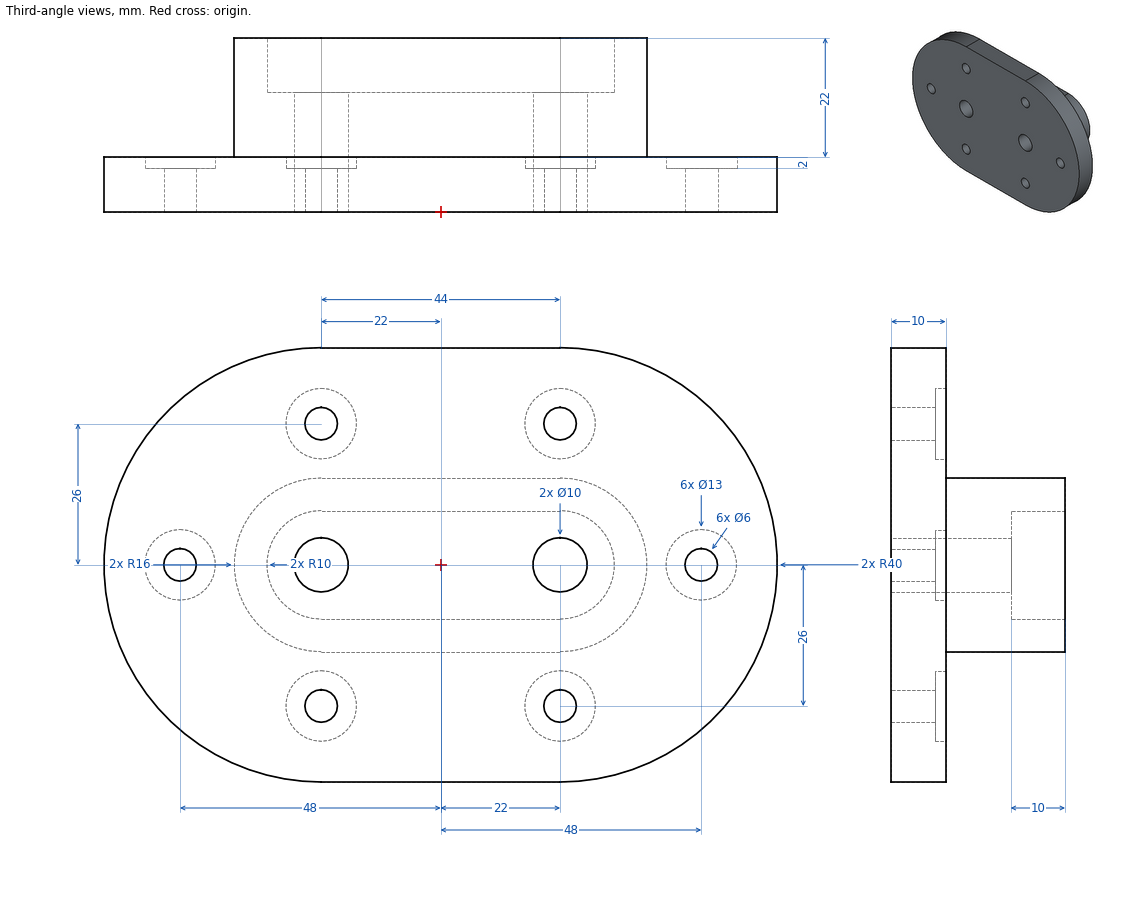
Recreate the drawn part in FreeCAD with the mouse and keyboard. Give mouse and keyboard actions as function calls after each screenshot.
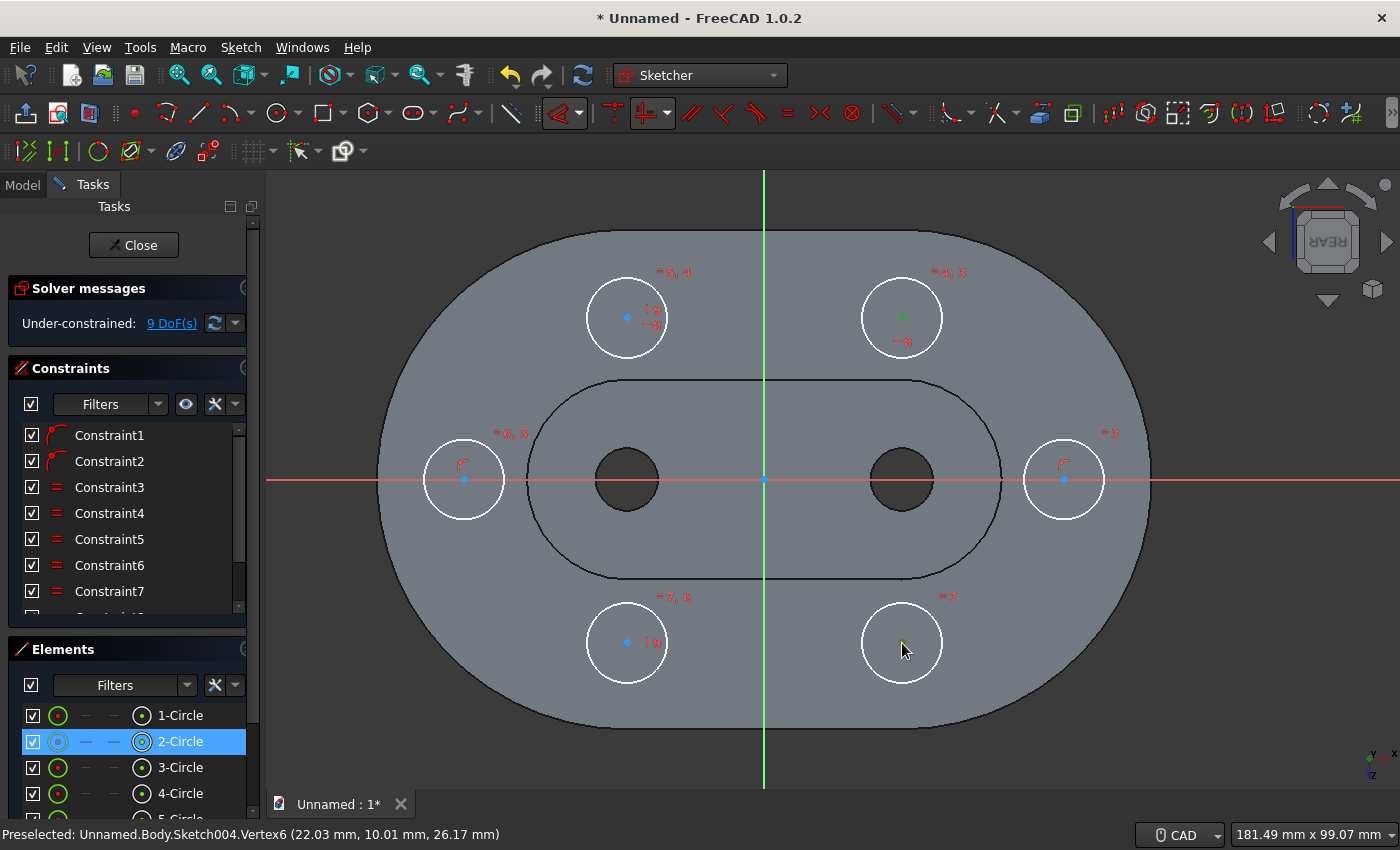
click(670, 114)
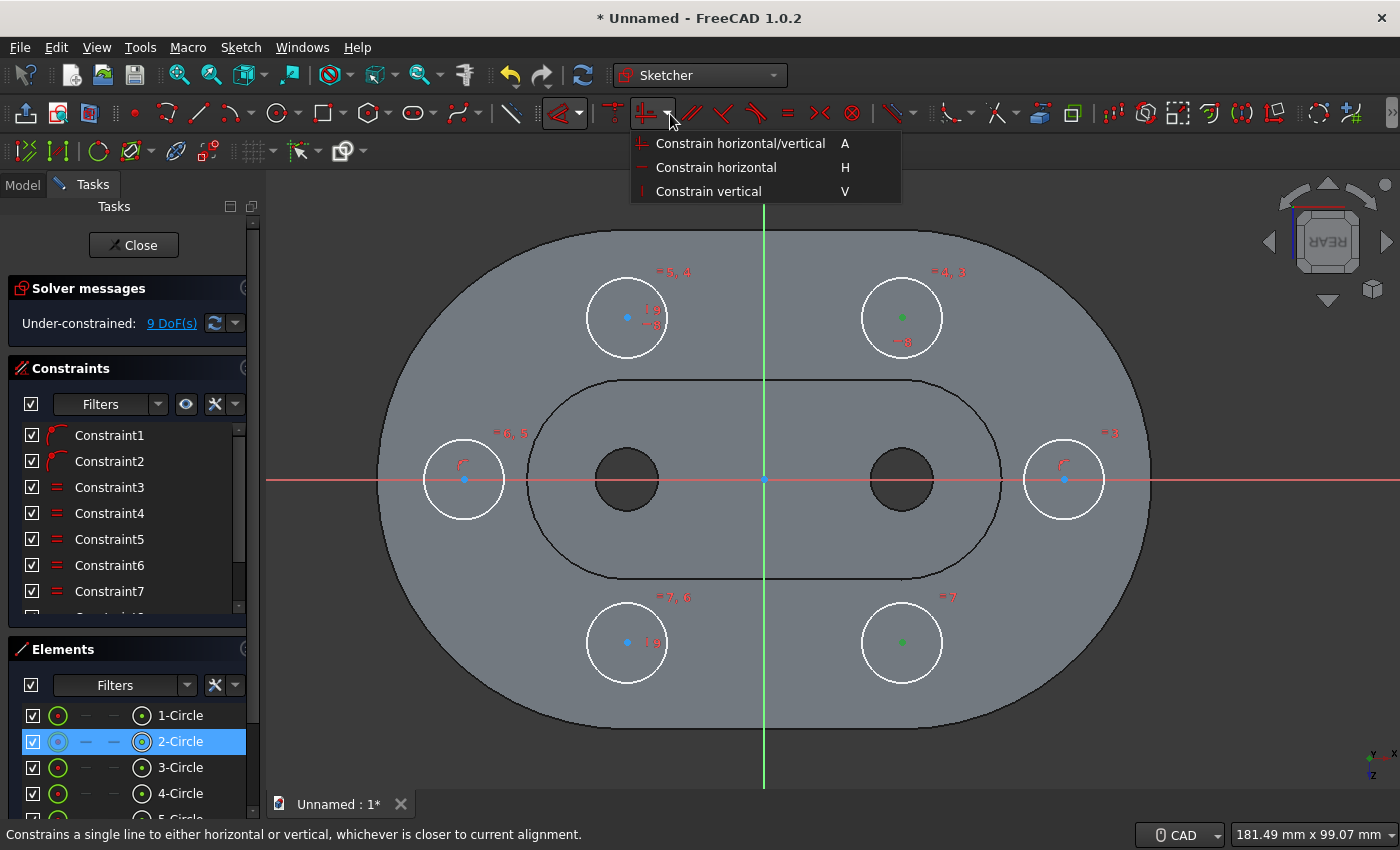
click(766, 191)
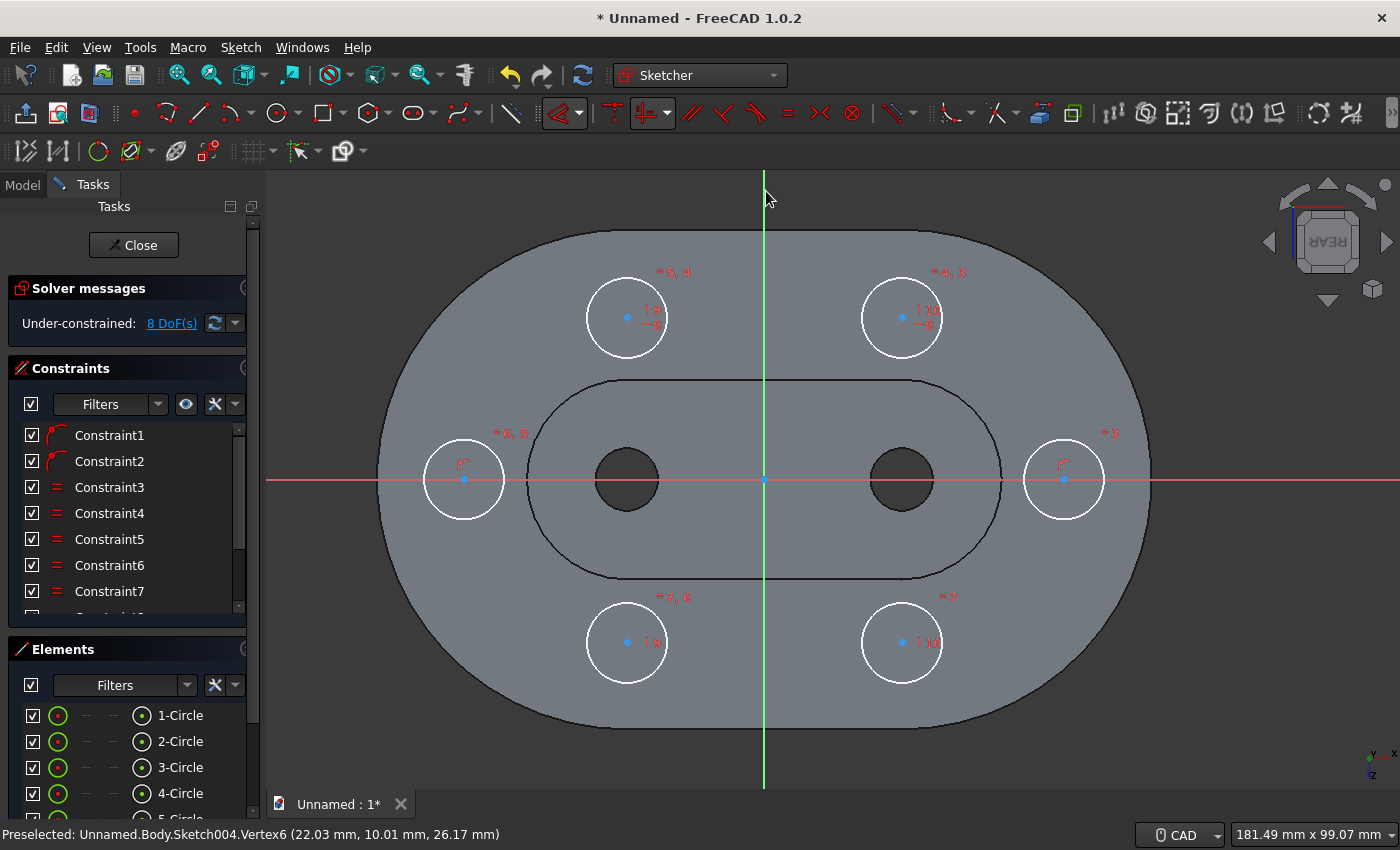
click(627, 643)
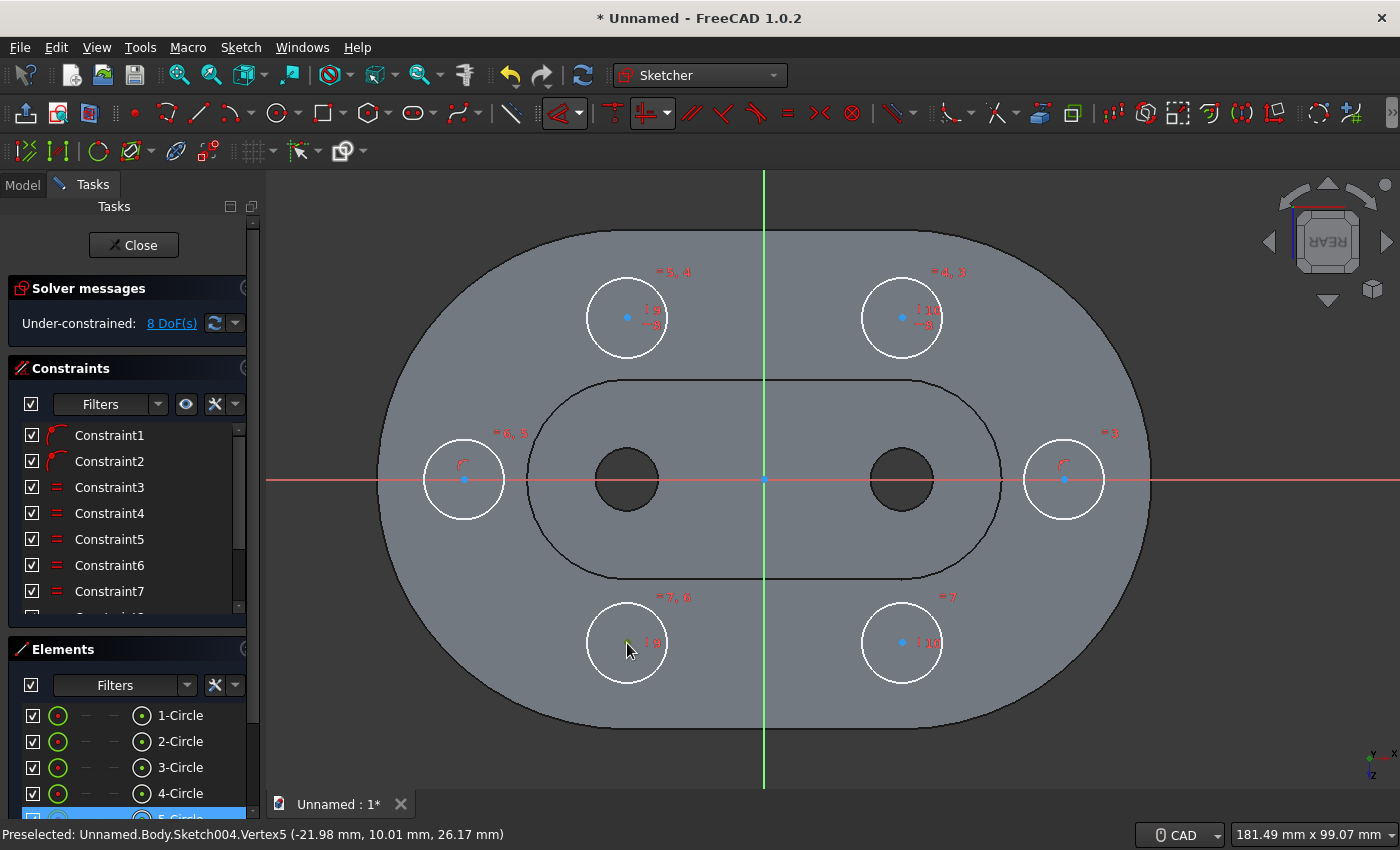
click(902, 643)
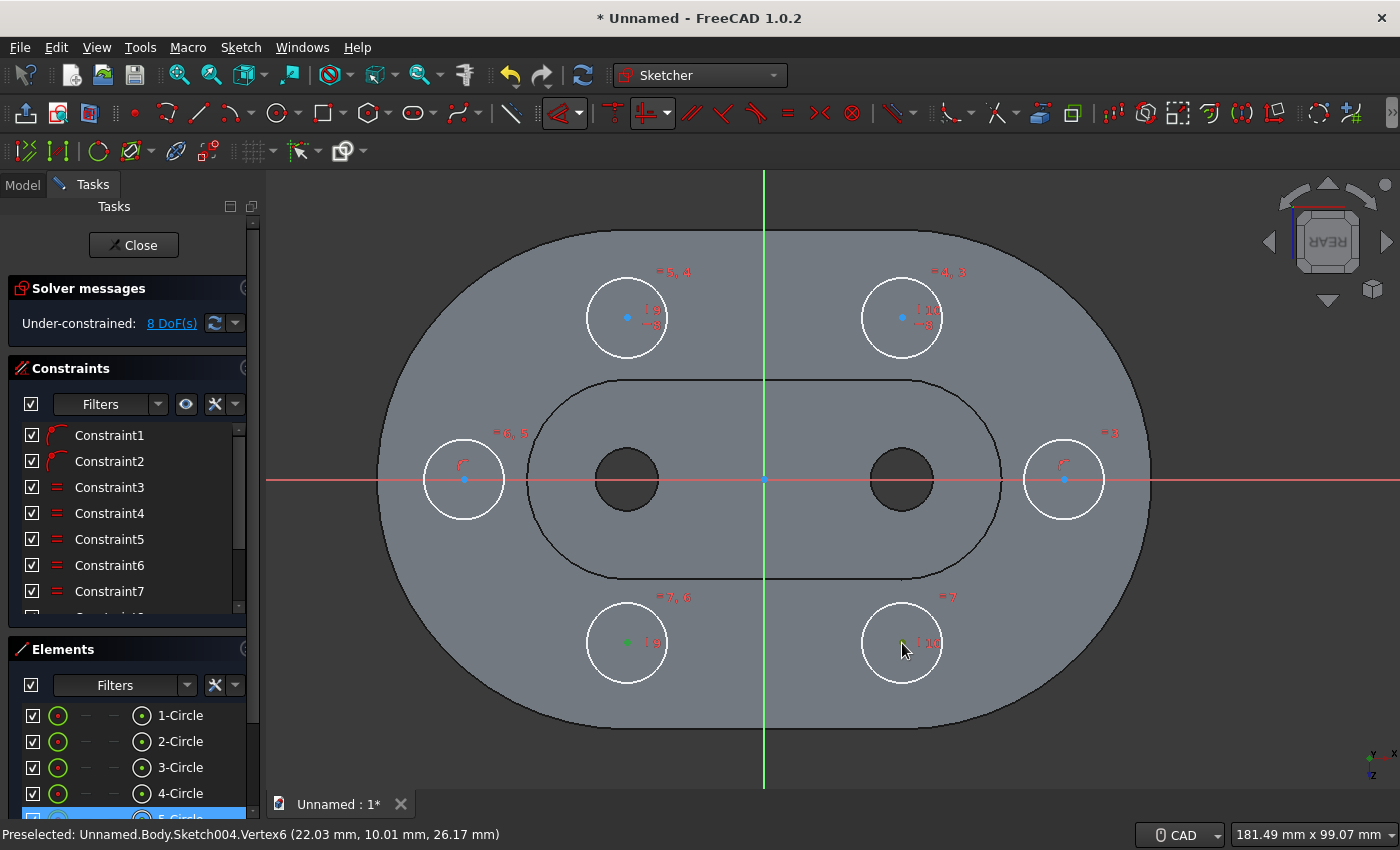
click(670, 114)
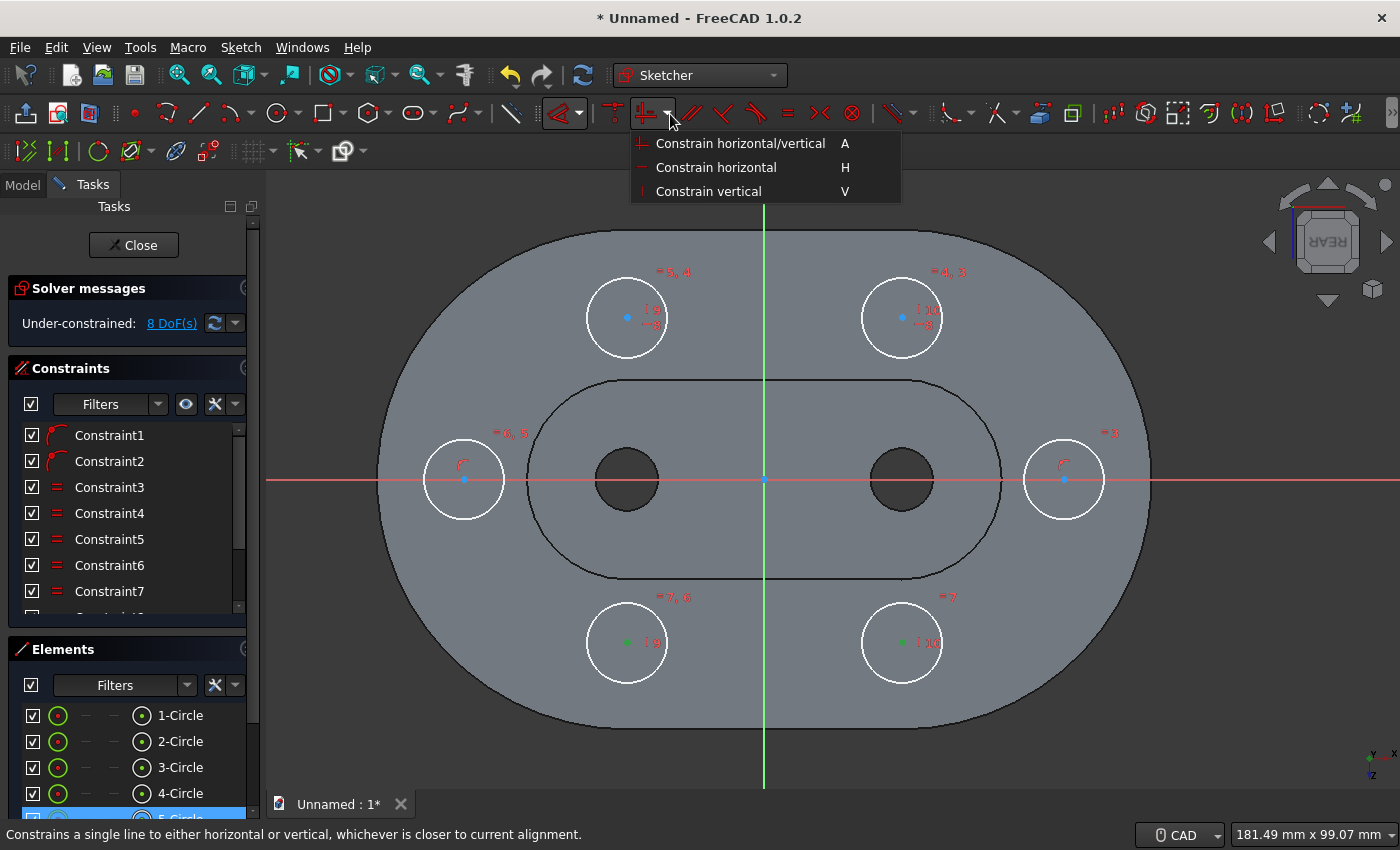
click(766, 167)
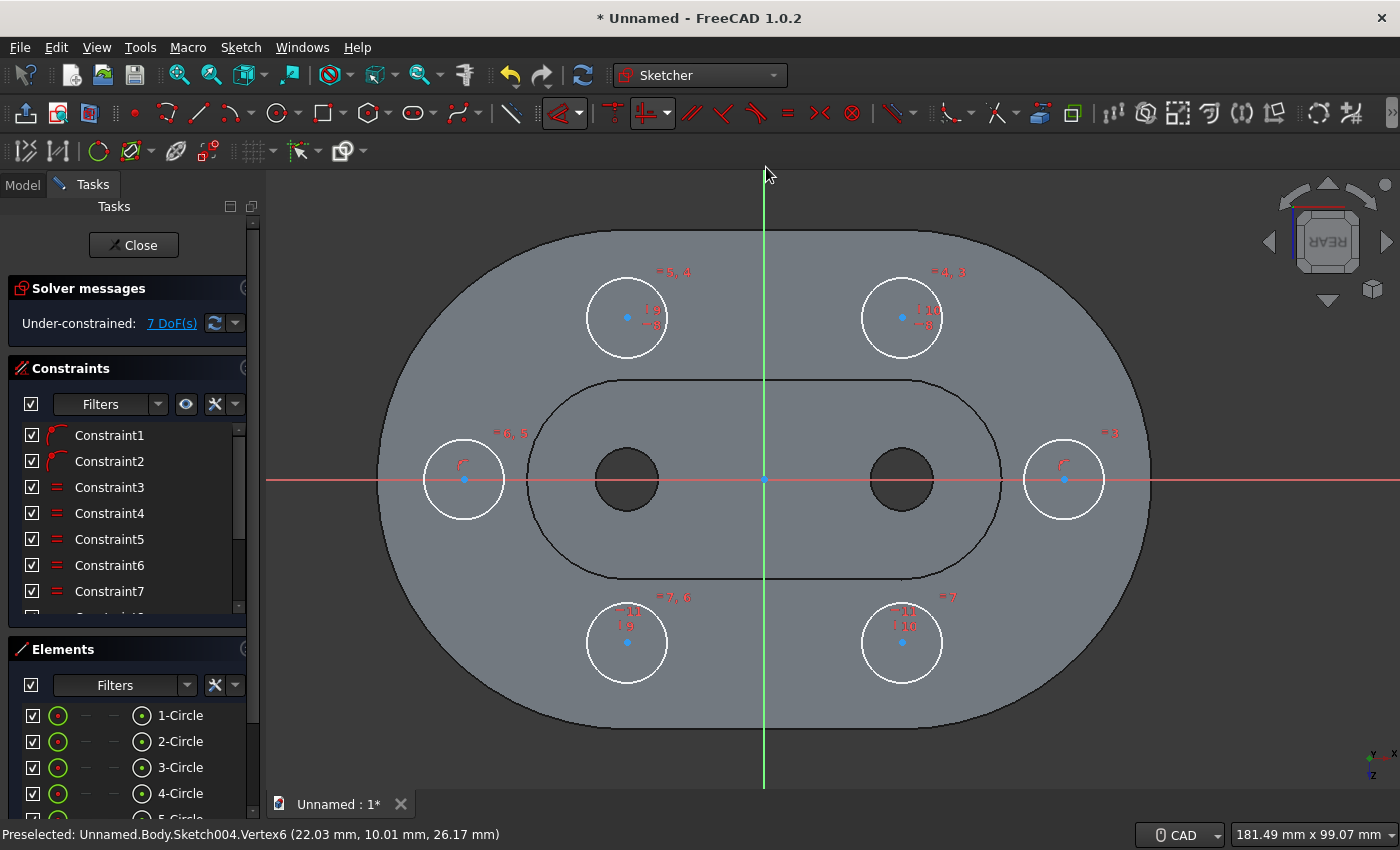
click(1092, 451)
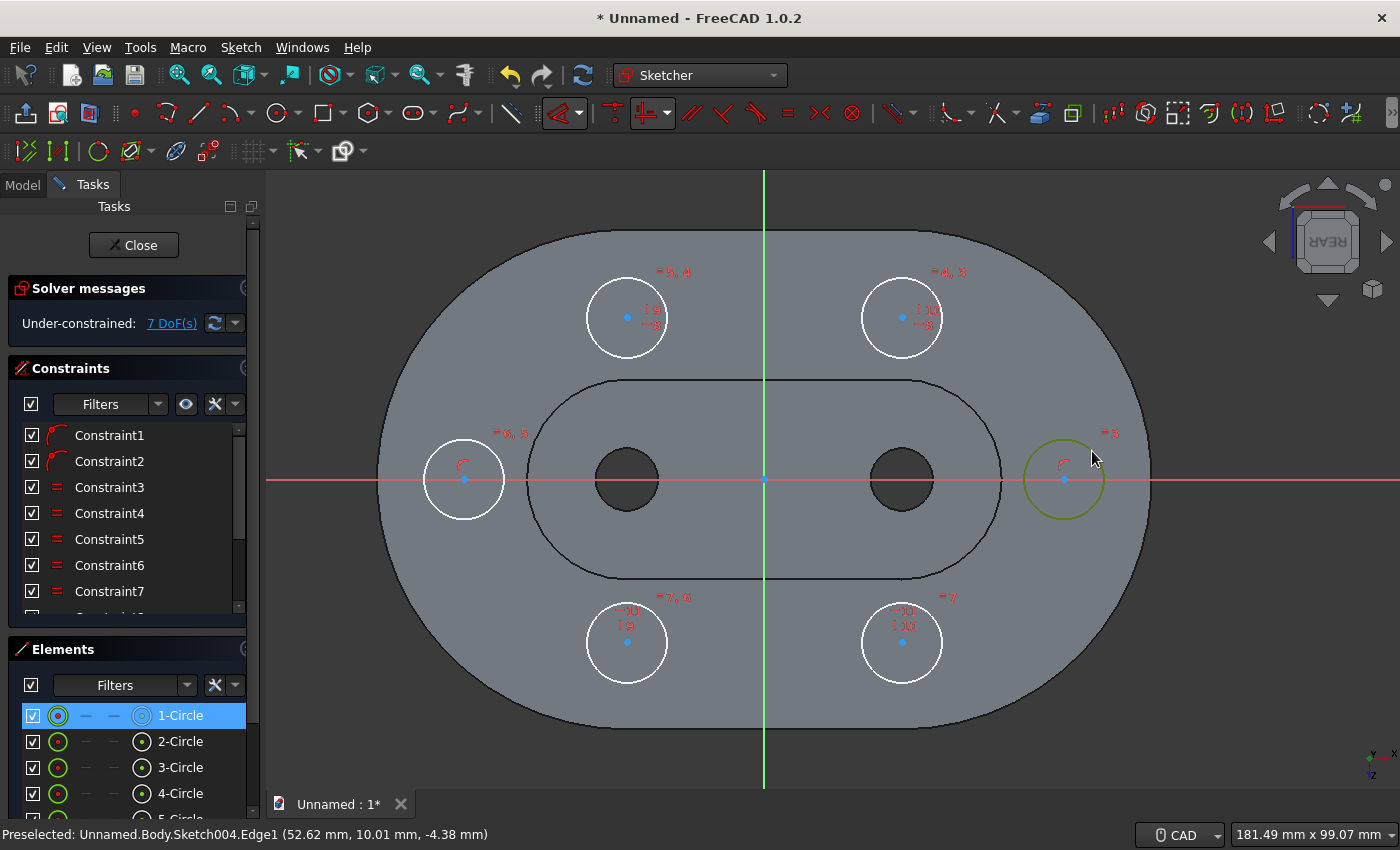
key(k)
key(o)